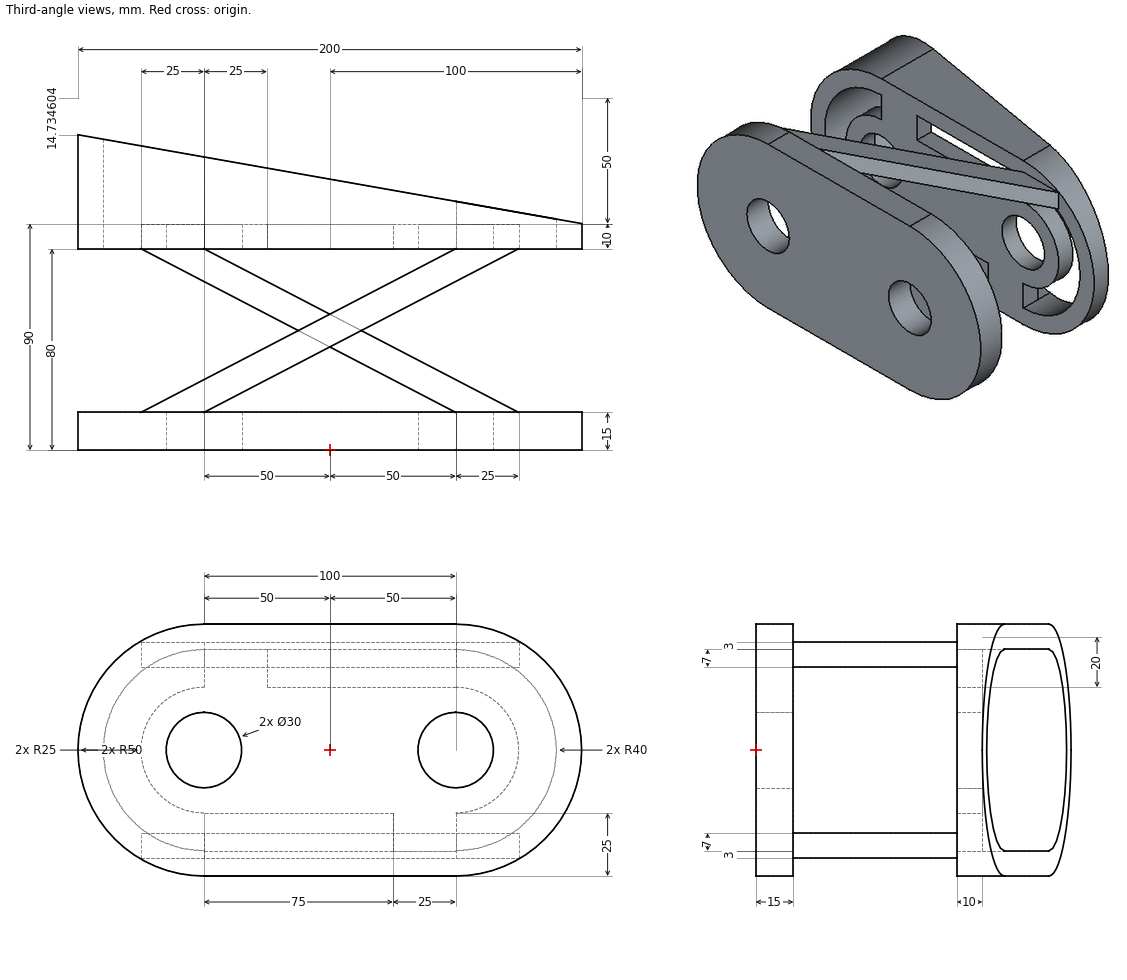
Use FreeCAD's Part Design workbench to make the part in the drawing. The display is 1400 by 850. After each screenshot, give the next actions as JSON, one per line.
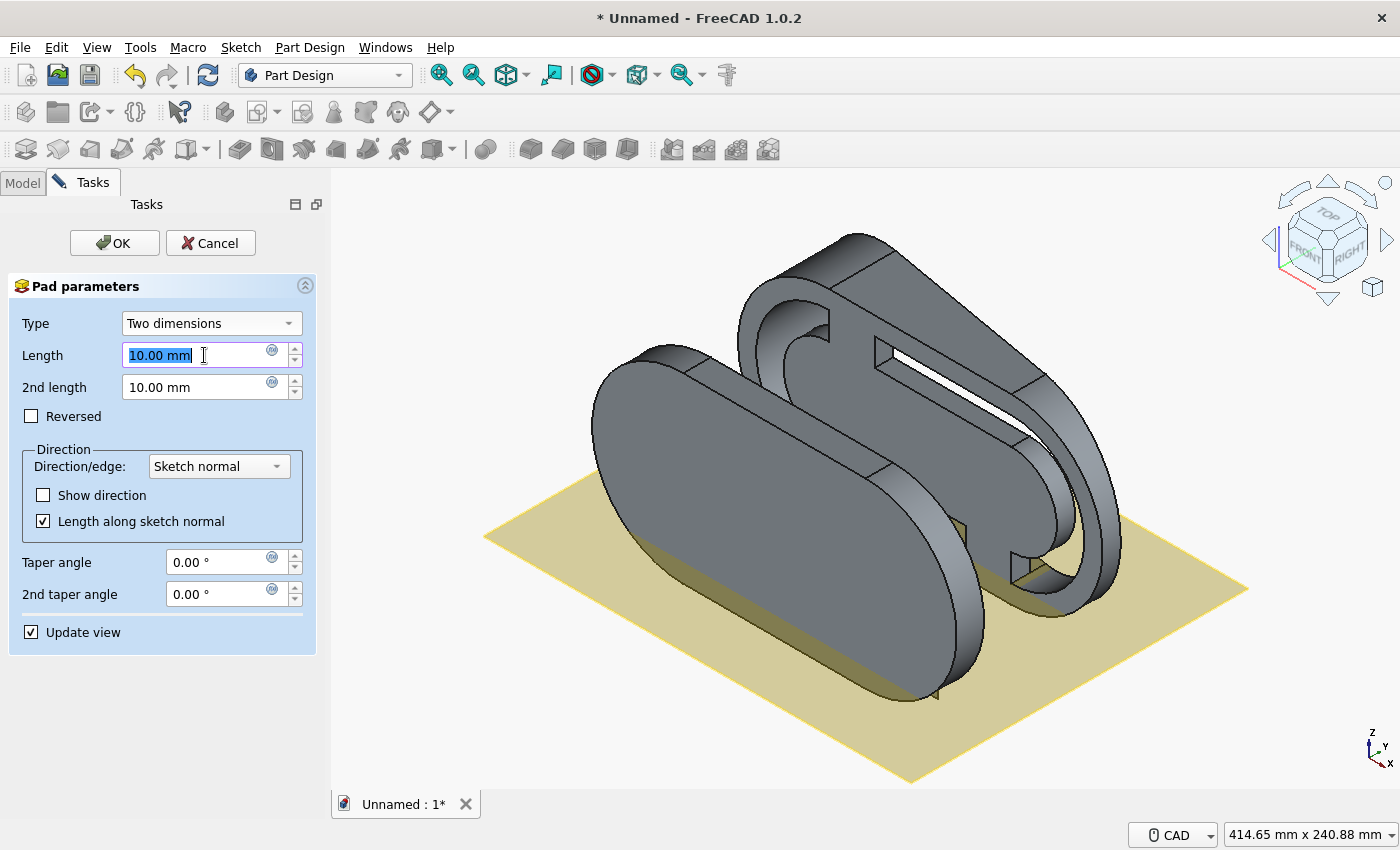
{"action": "type", "text": "7"}
{"action": "key", "text": "Tab"}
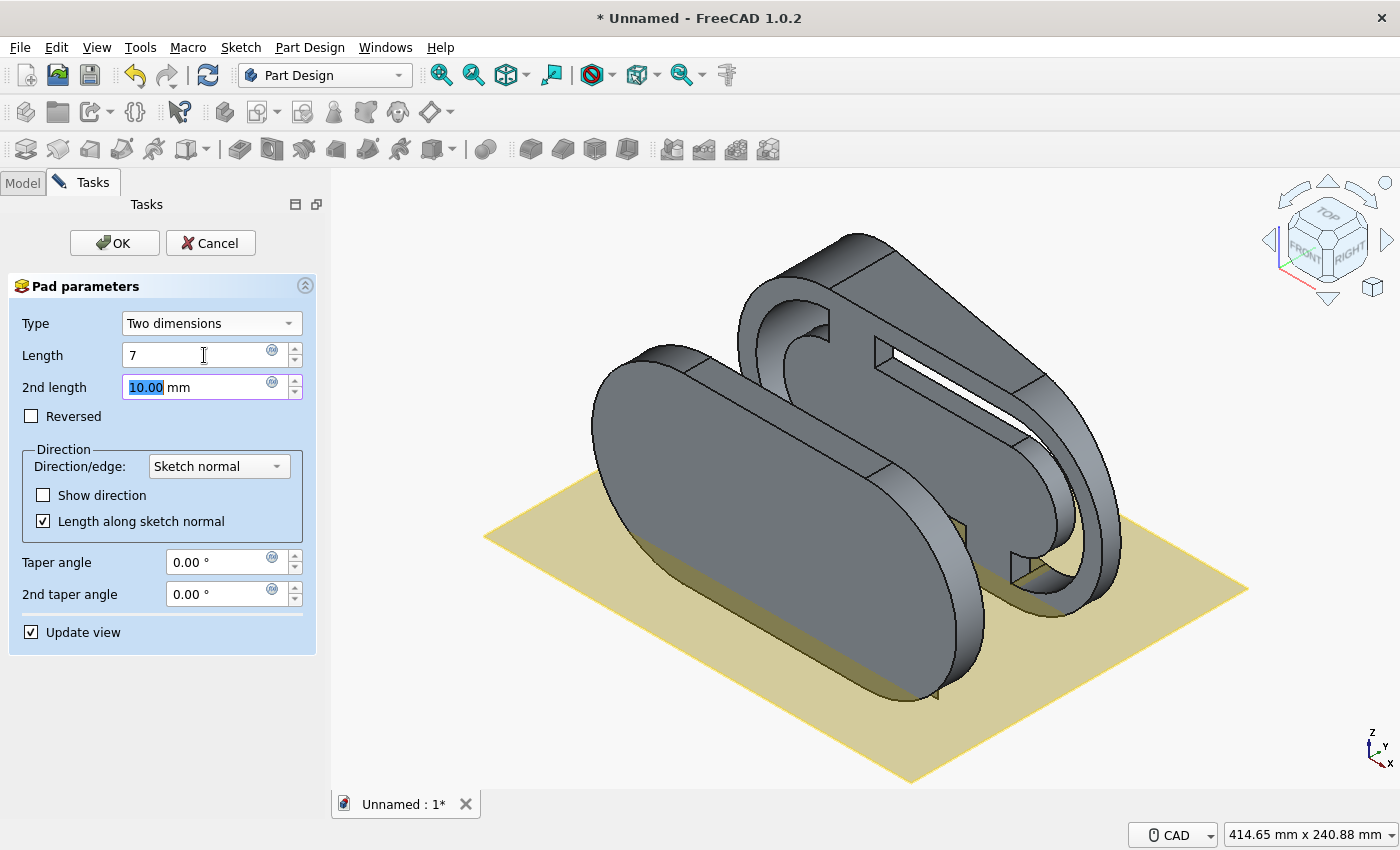
{"action": "type", "text": "3"}
{"action": "key", "text": "Tab"}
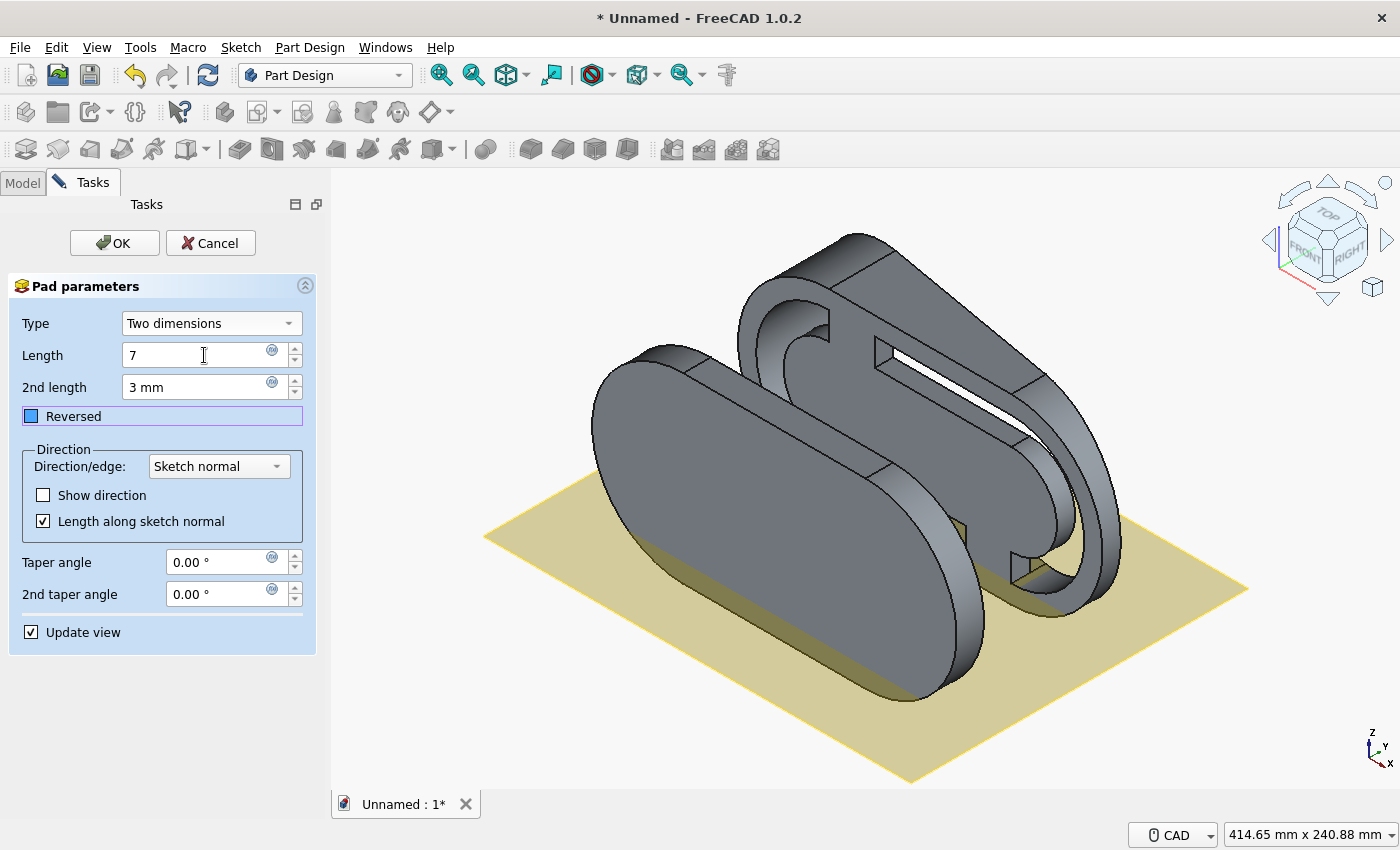
{"action": "left_click", "coordinate": [115, 243]}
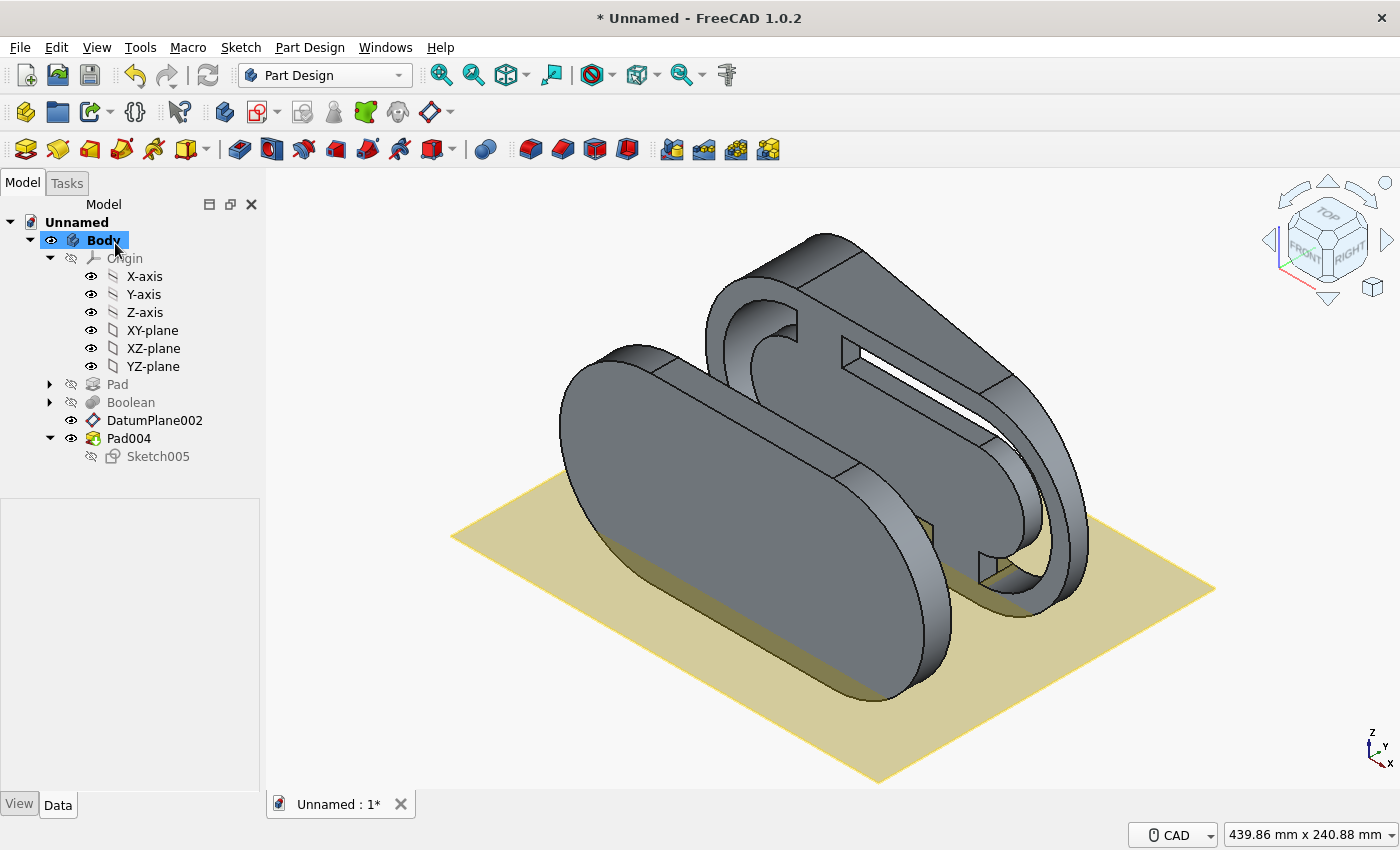
{"action": "left_click", "coordinate": [116, 420]}
{"action": "key", "text": "space"}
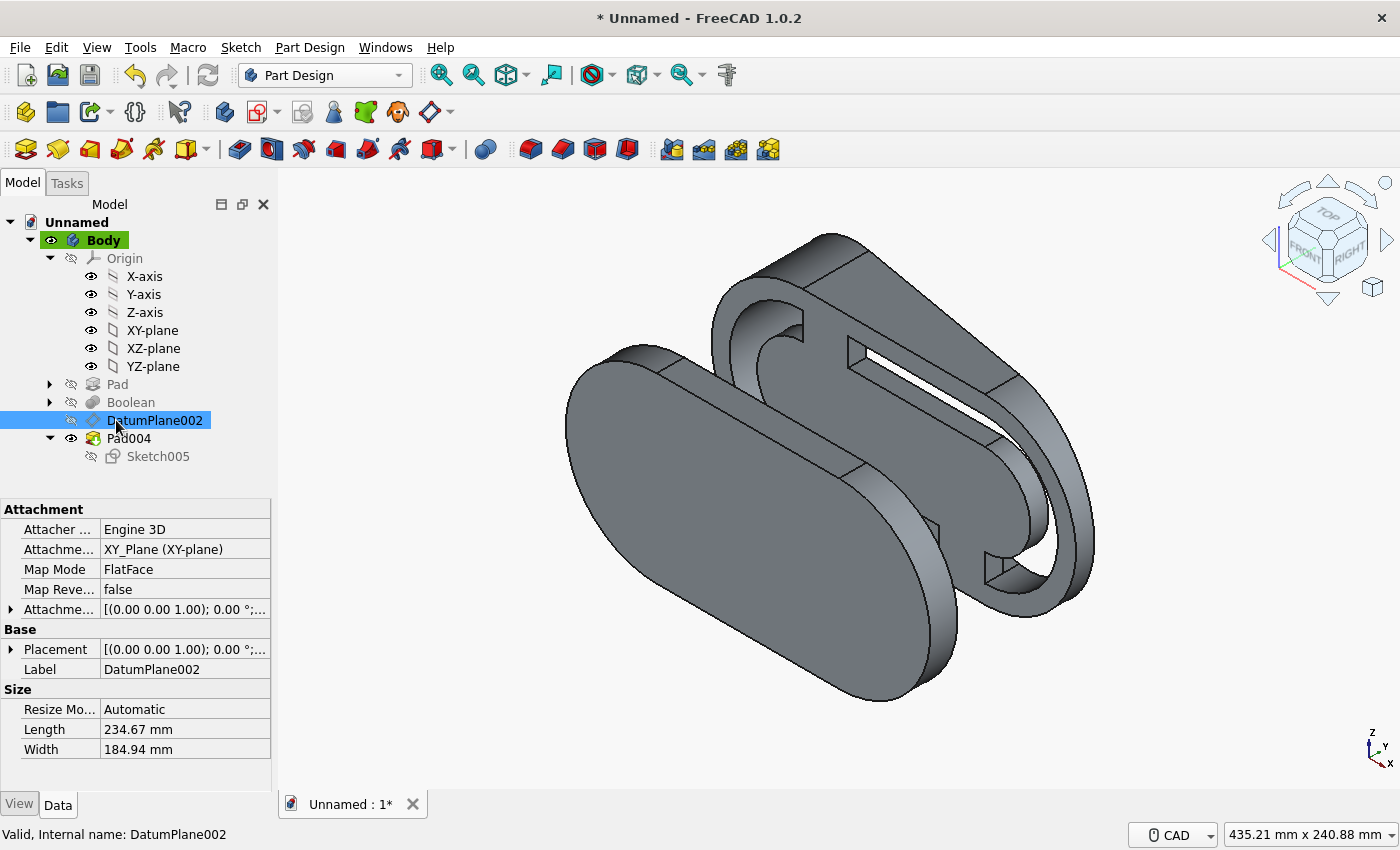
{"action": "left_click", "coordinate": [136, 330]}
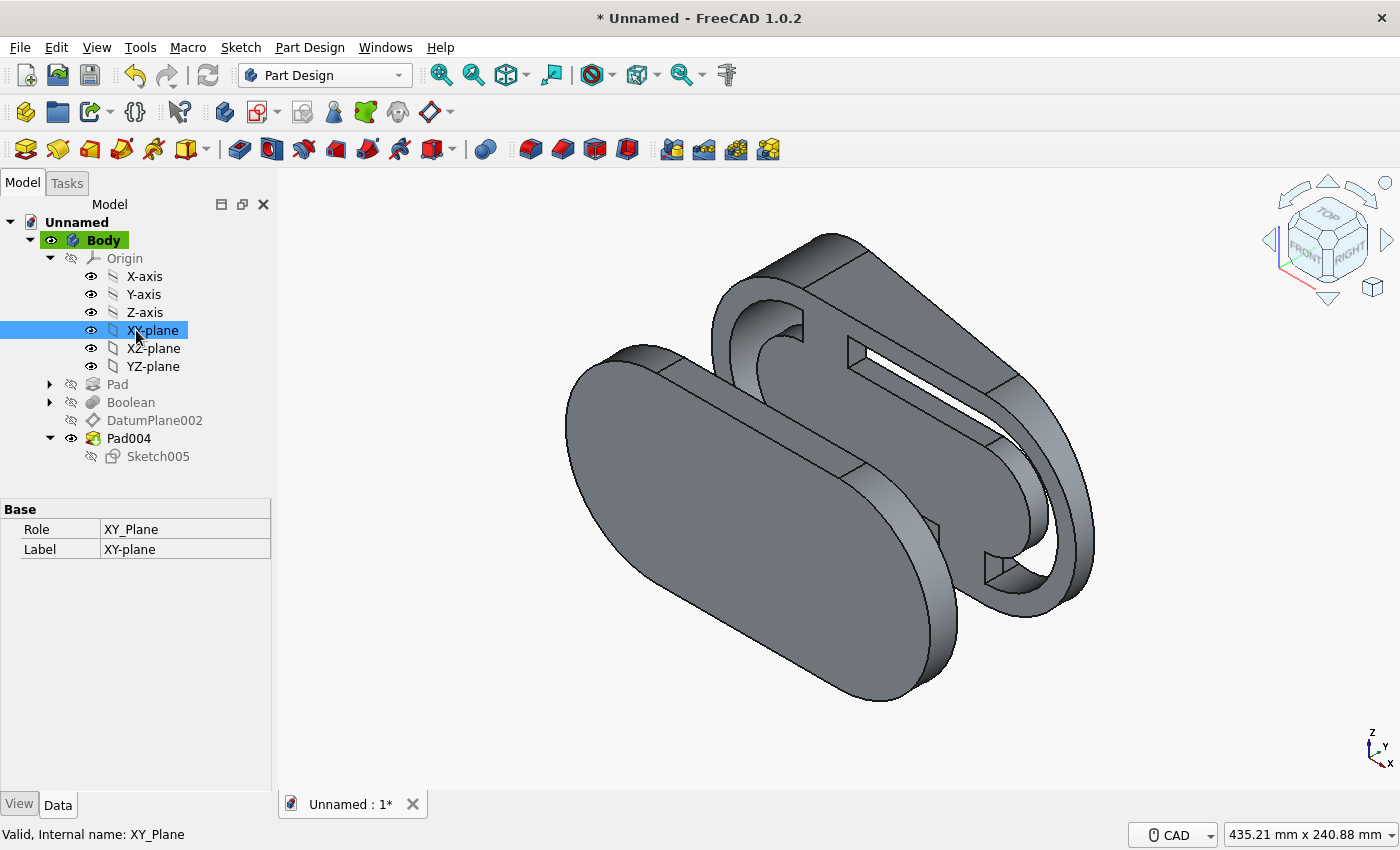
{"action": "left_click", "coordinate": [430, 112]}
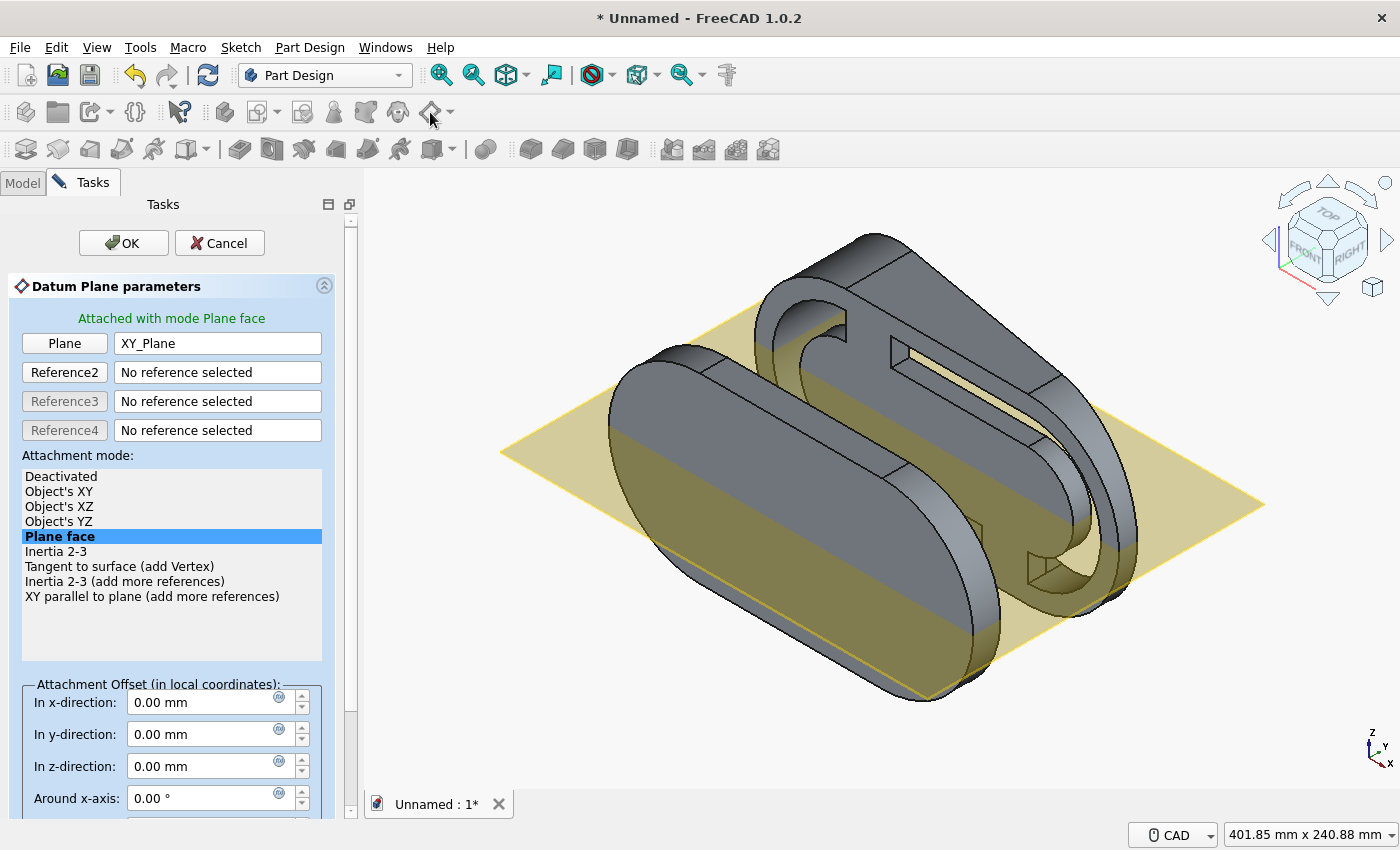
{"action": "triple_click", "coordinate": [210, 766]}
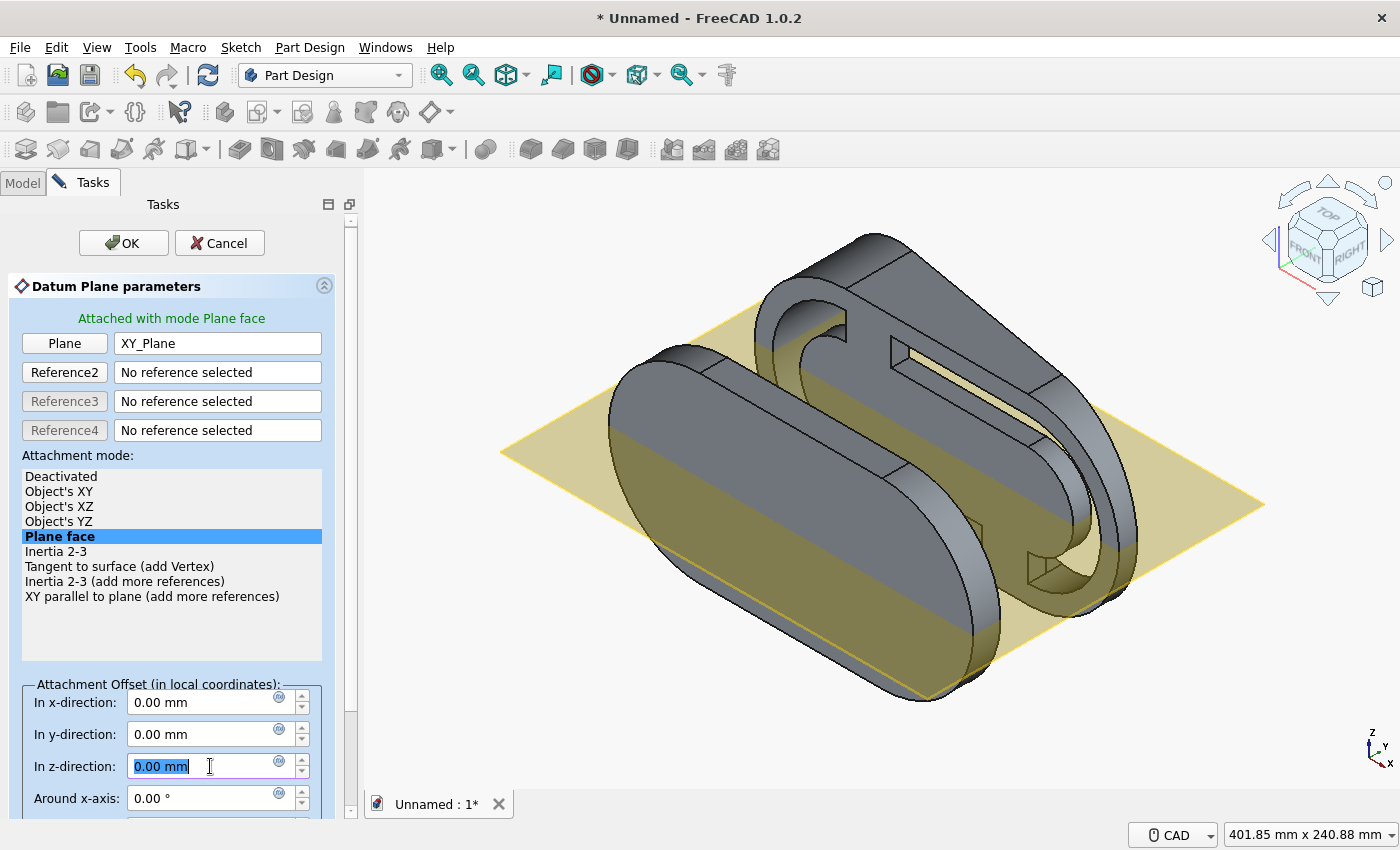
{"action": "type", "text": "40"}
{"action": "key", "text": "Tab"}